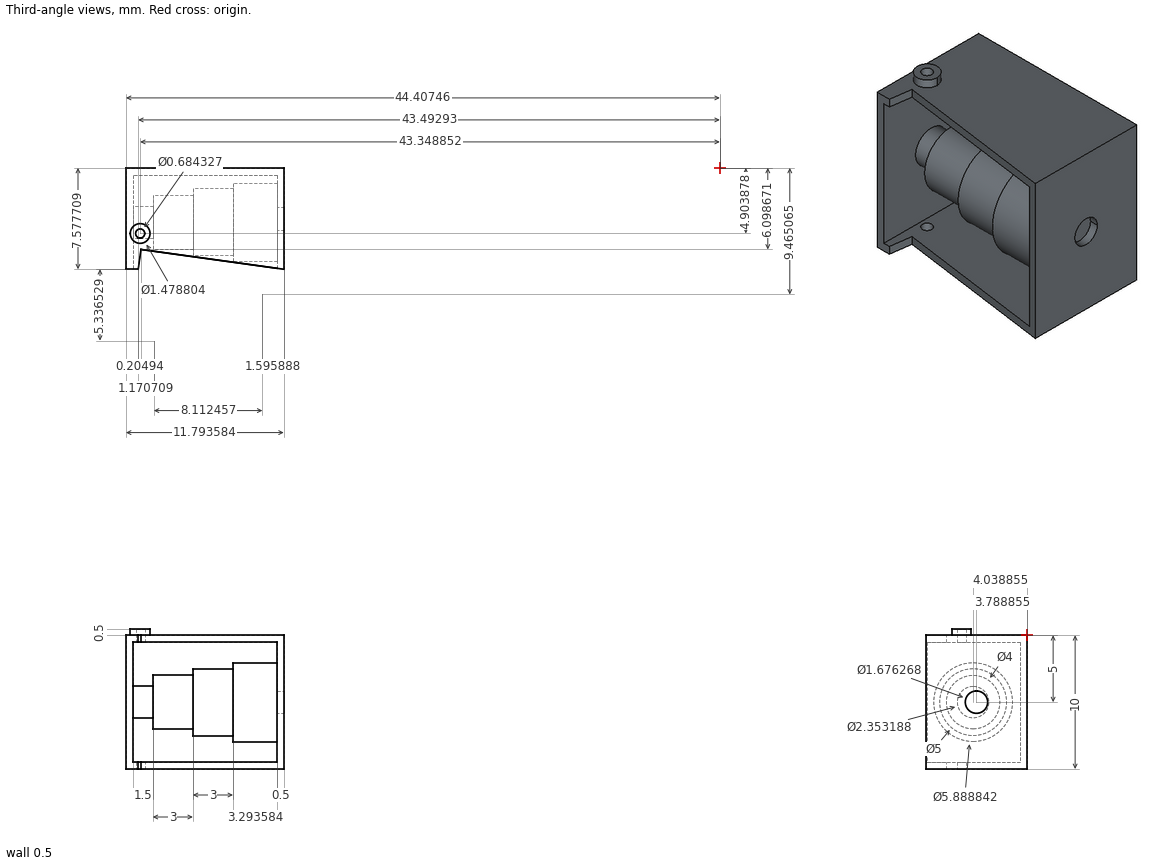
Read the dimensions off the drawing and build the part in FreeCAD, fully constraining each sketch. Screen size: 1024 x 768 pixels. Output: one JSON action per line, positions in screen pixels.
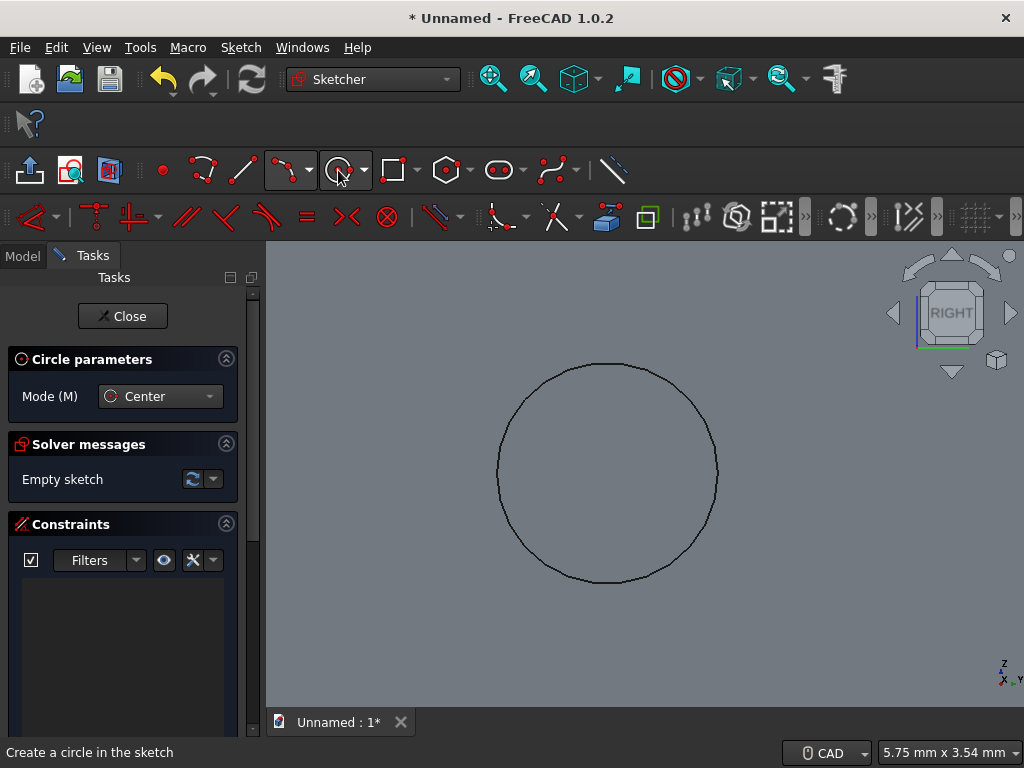
{"action": "left_click", "coordinate": [574, 473]}
{"action": "left_click", "coordinate": [684, 364]}
{"action": "key", "text": "Escape"}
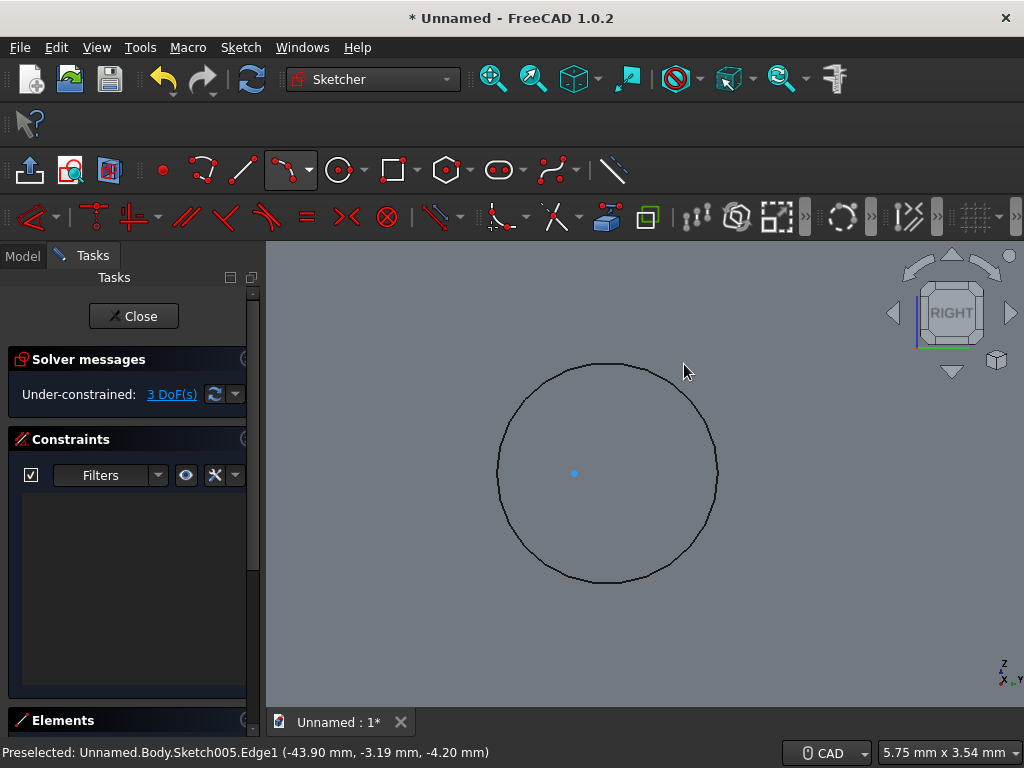
{"action": "left_click", "coordinate": [32, 218]}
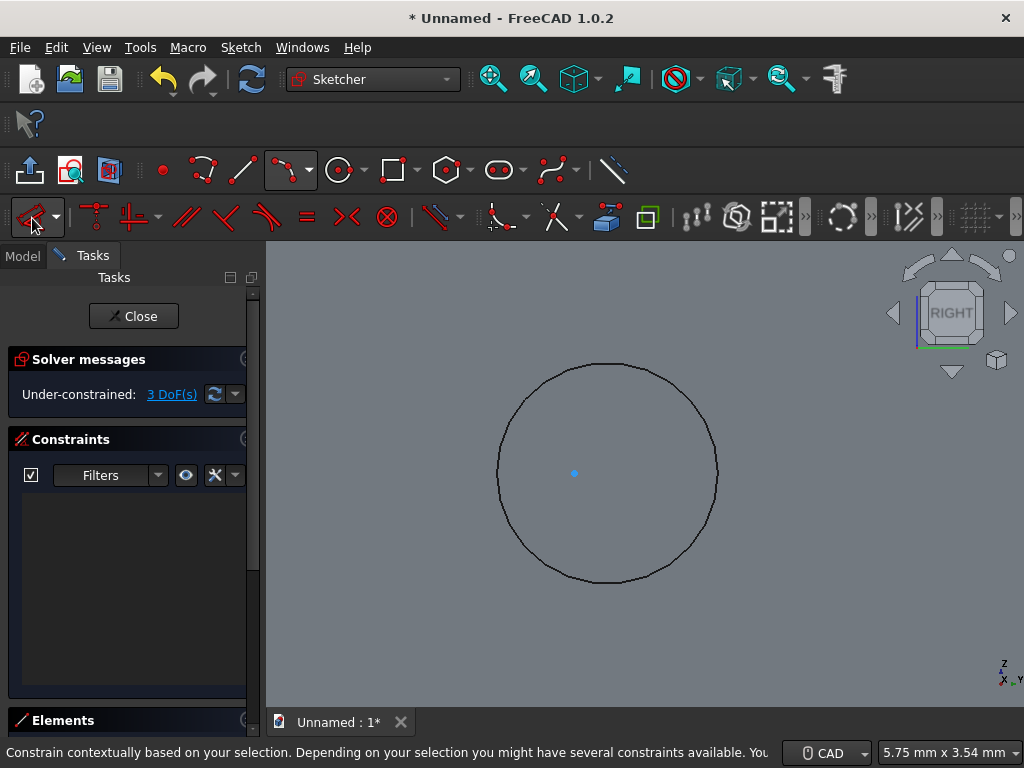
{"action": "left_click", "coordinate": [683, 364]}
{"action": "left_click", "coordinate": [706, 341]}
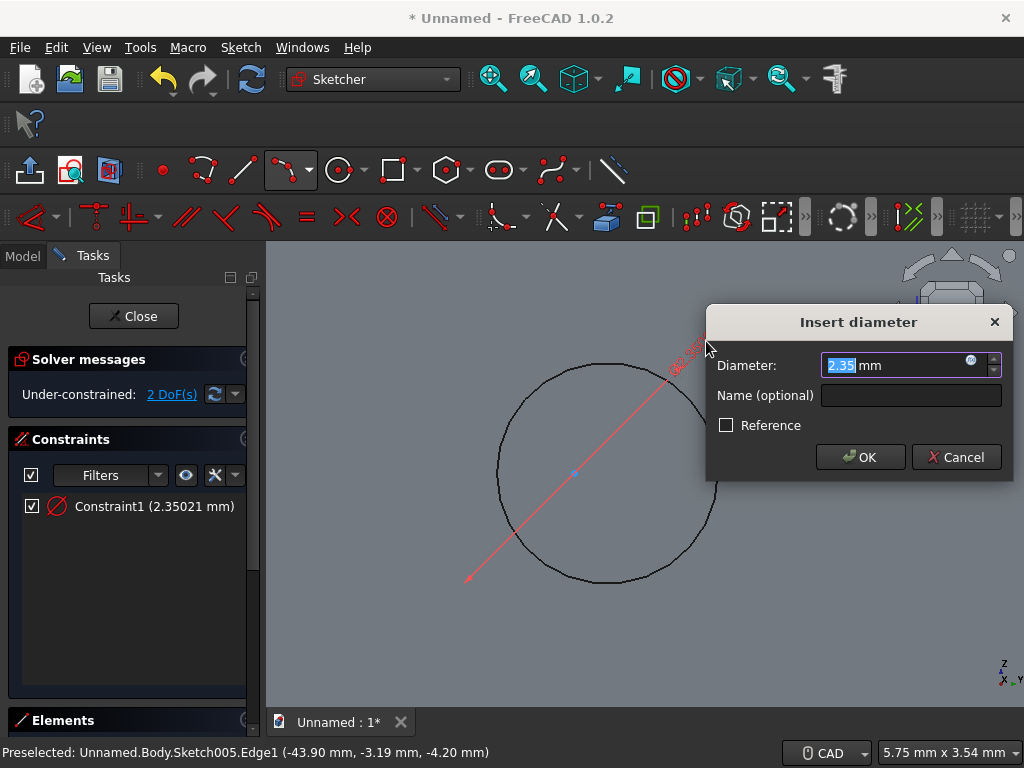
{"action": "type", "text": "2.353188"}
{"action": "key", "text": "Return"}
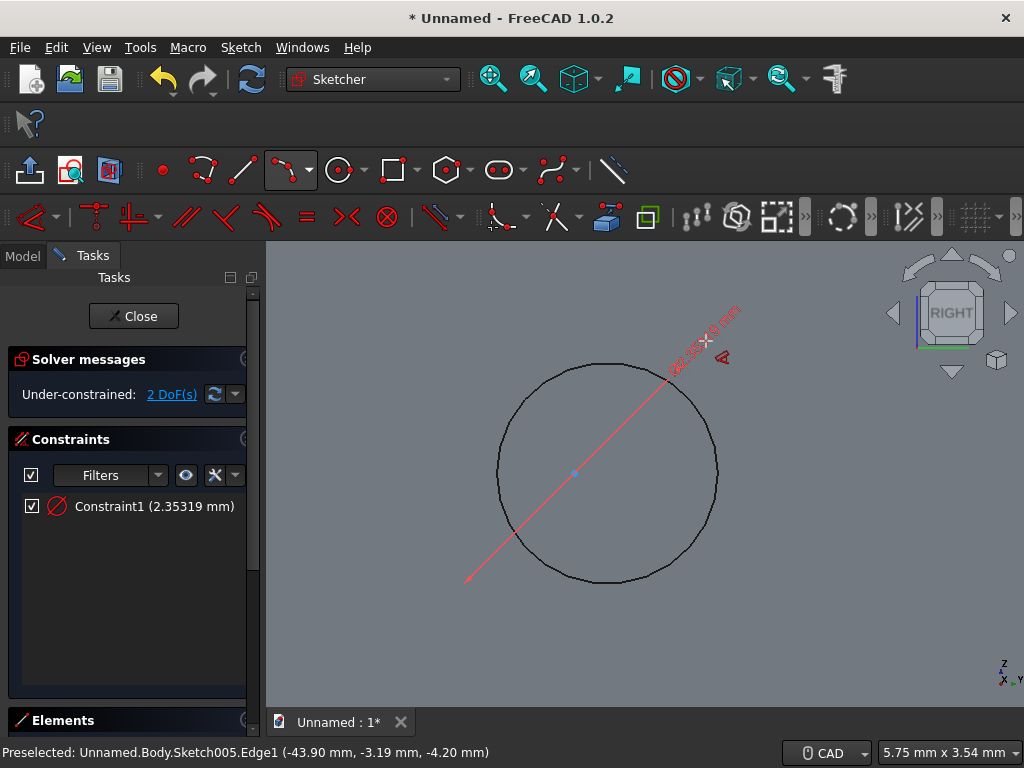
{"action": "left_click", "coordinate": [574, 474]}
{"action": "left_click", "coordinate": [540, 372]}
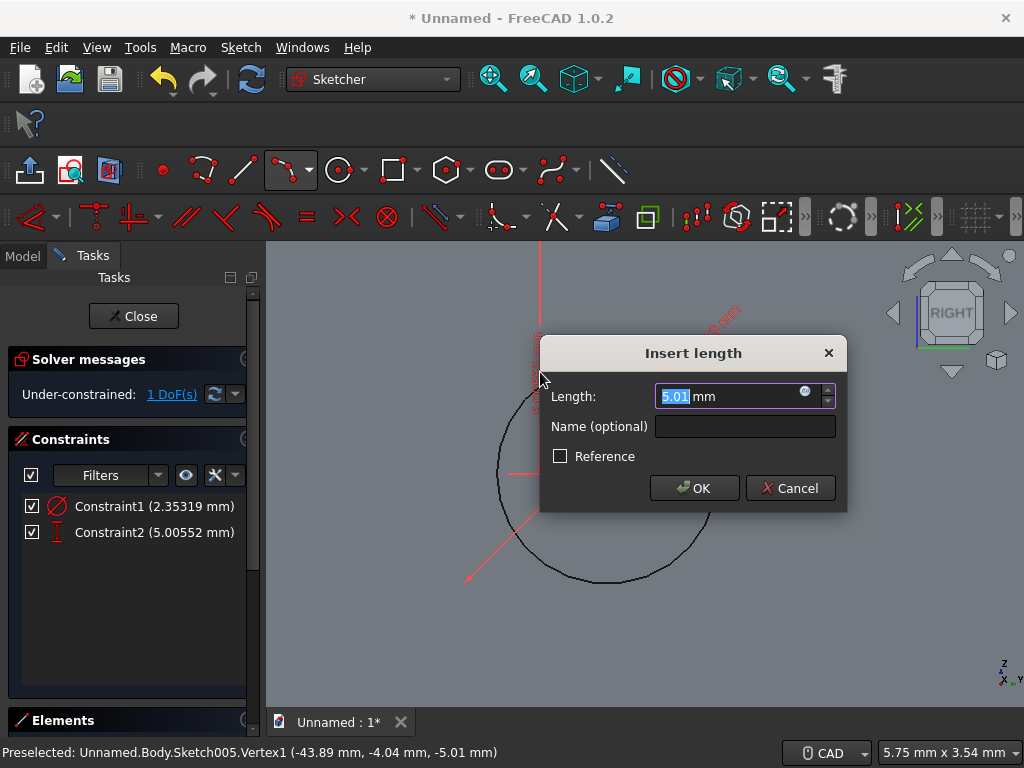
{"action": "type", "text": "5"}
{"action": "key", "text": "Return"}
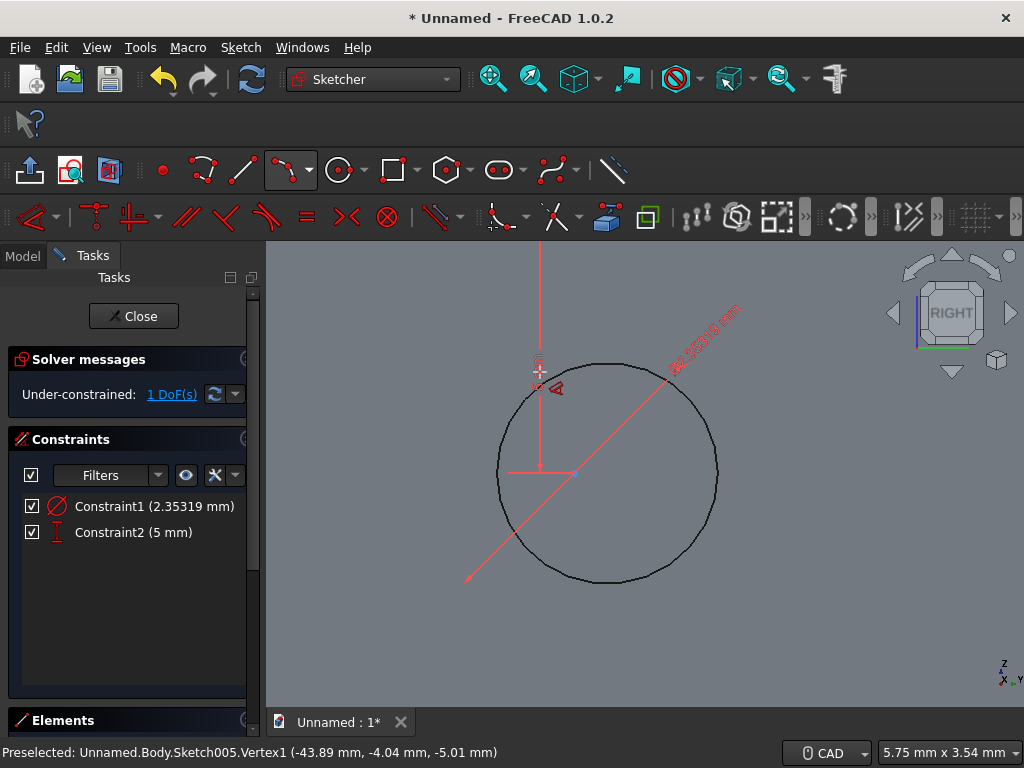
{"action": "left_click", "coordinate": [574, 473]}
{"action": "left_click", "coordinate": [651, 507]}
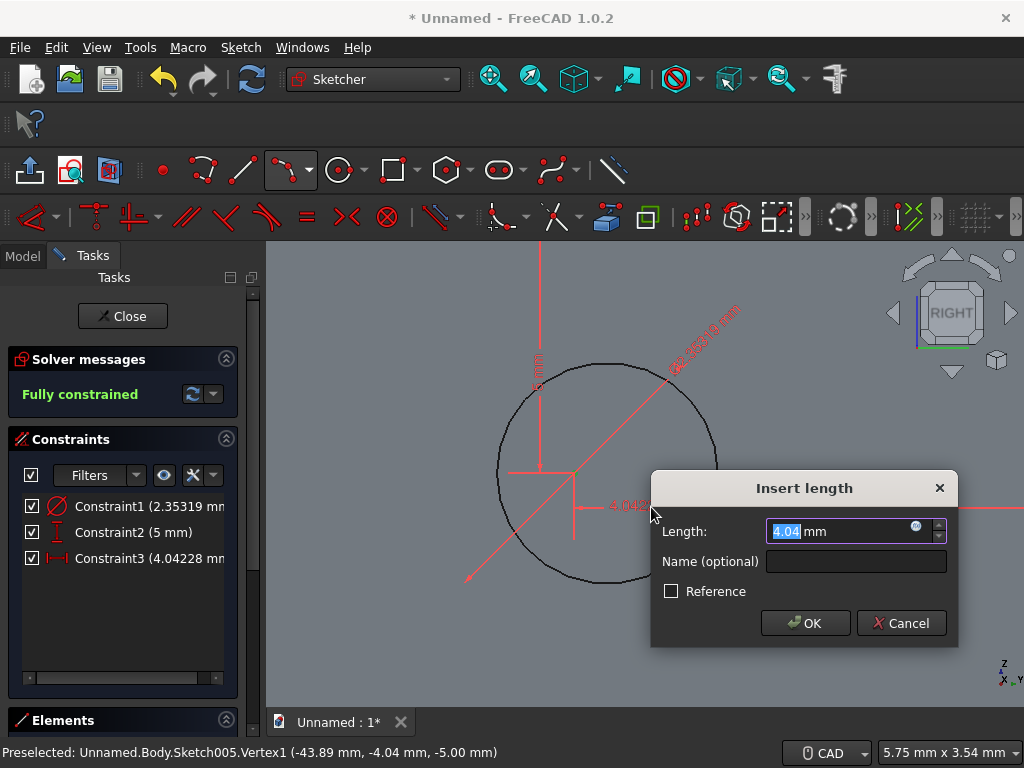
{"action": "type", "text": "4.038855"}
{"action": "key", "text": "Return"}
{"action": "key", "text": "Escape"}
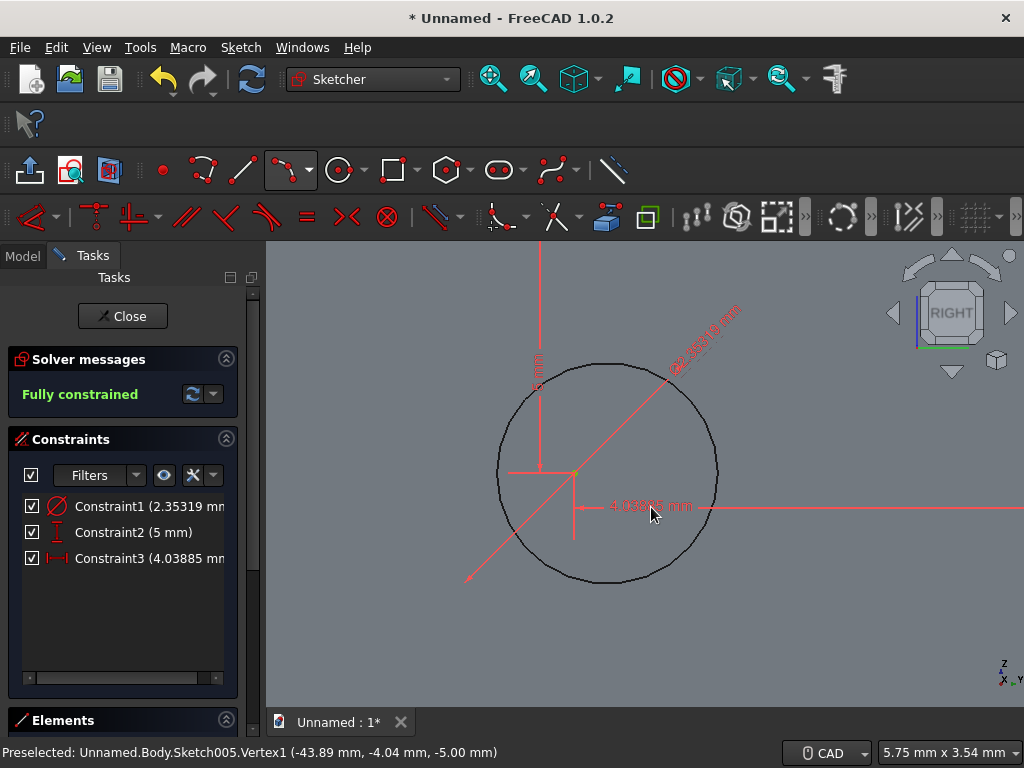
{"action": "left_click", "coordinate": [123, 316]}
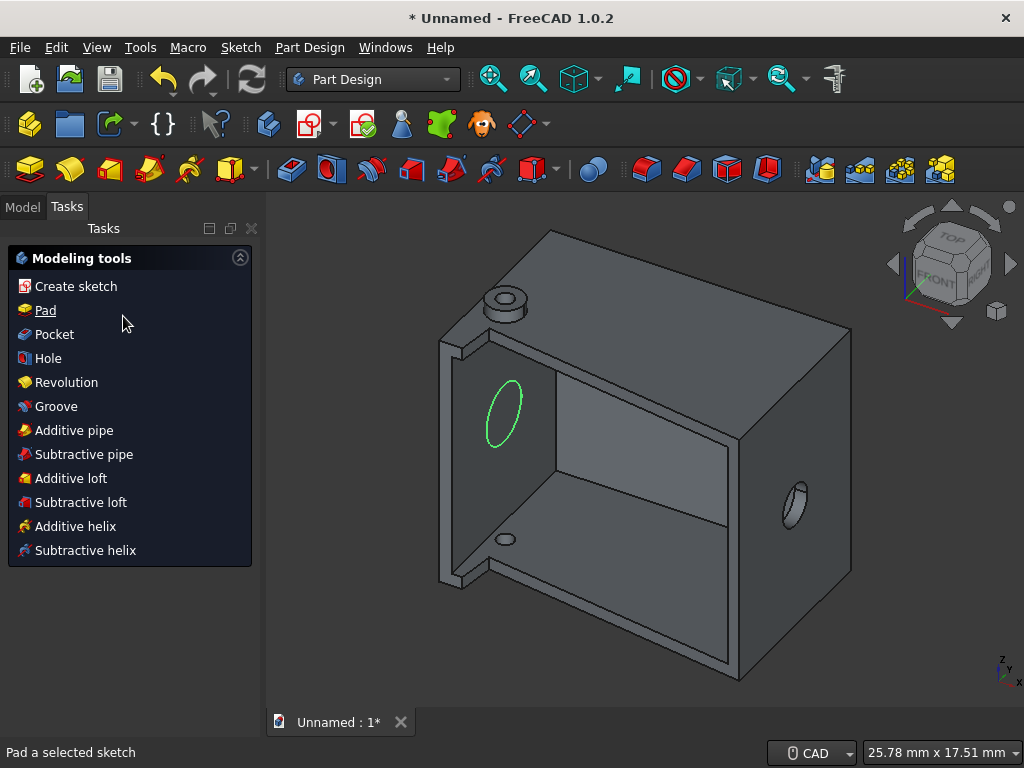
{"action": "left_click", "coordinate": [30, 170]}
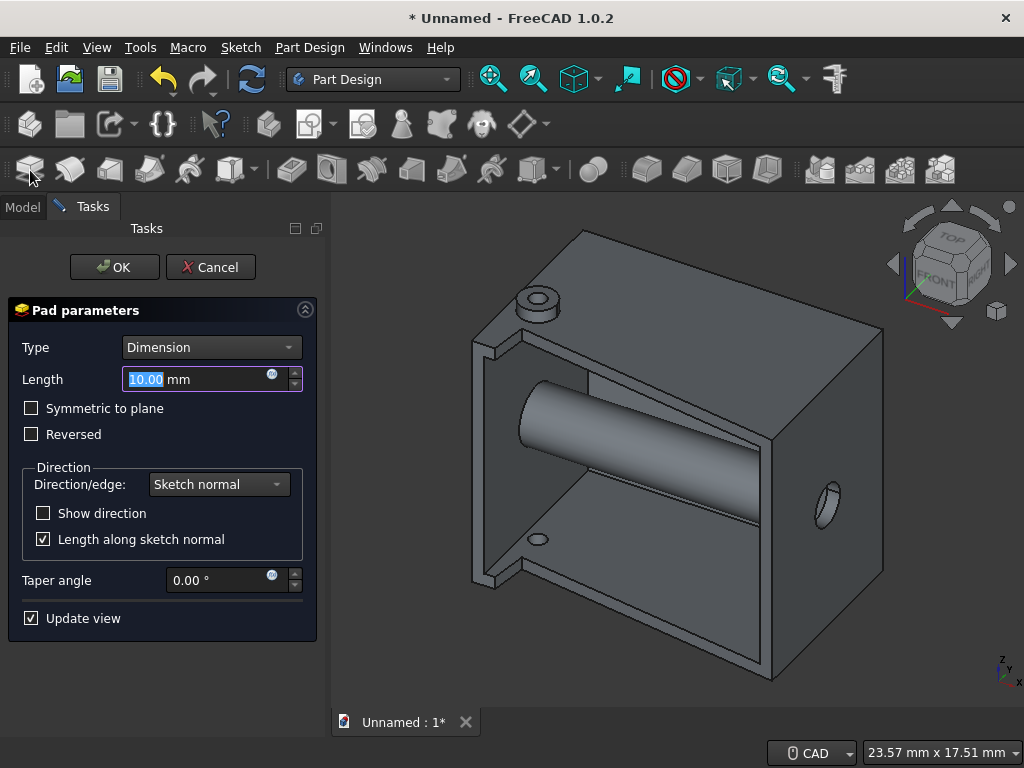
{"action": "type", "text": "1.5"}
{"action": "key", "text": "Tab"}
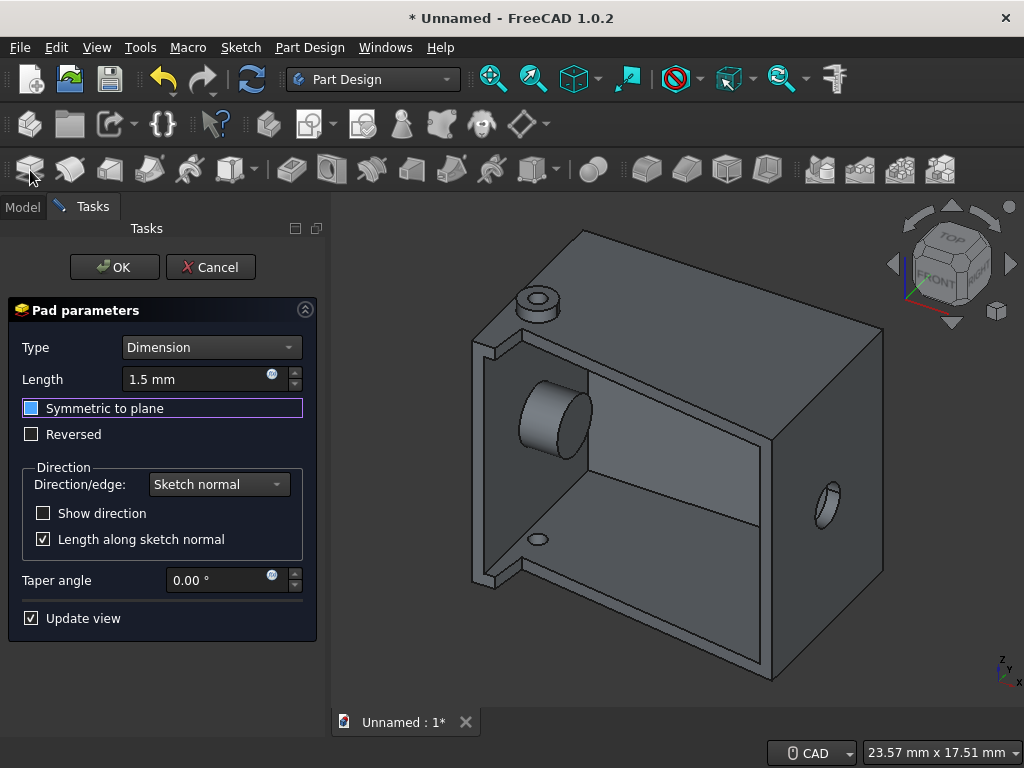
{"action": "left_click", "coordinate": [115, 267]}